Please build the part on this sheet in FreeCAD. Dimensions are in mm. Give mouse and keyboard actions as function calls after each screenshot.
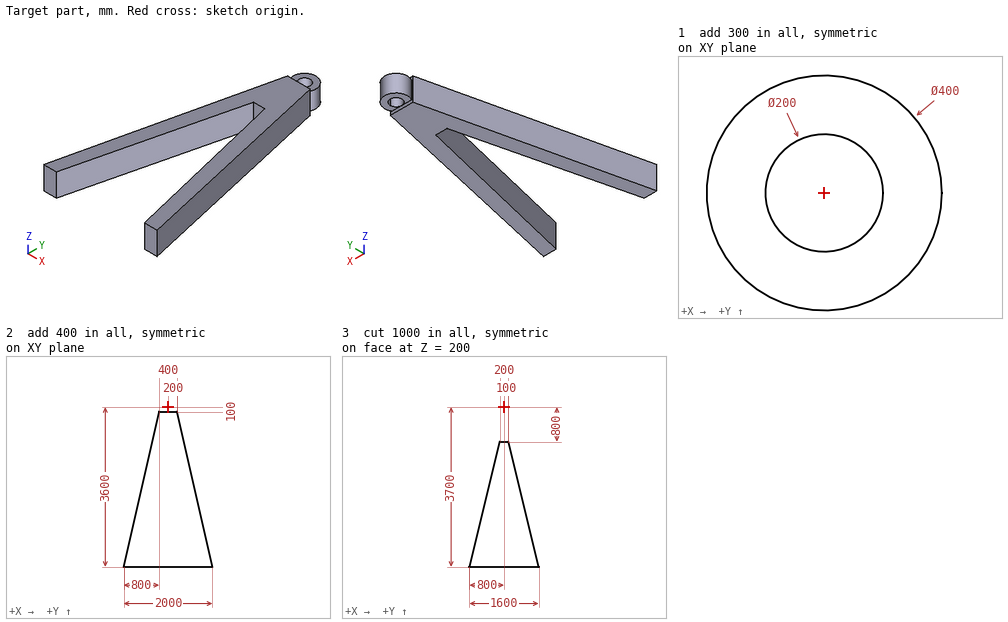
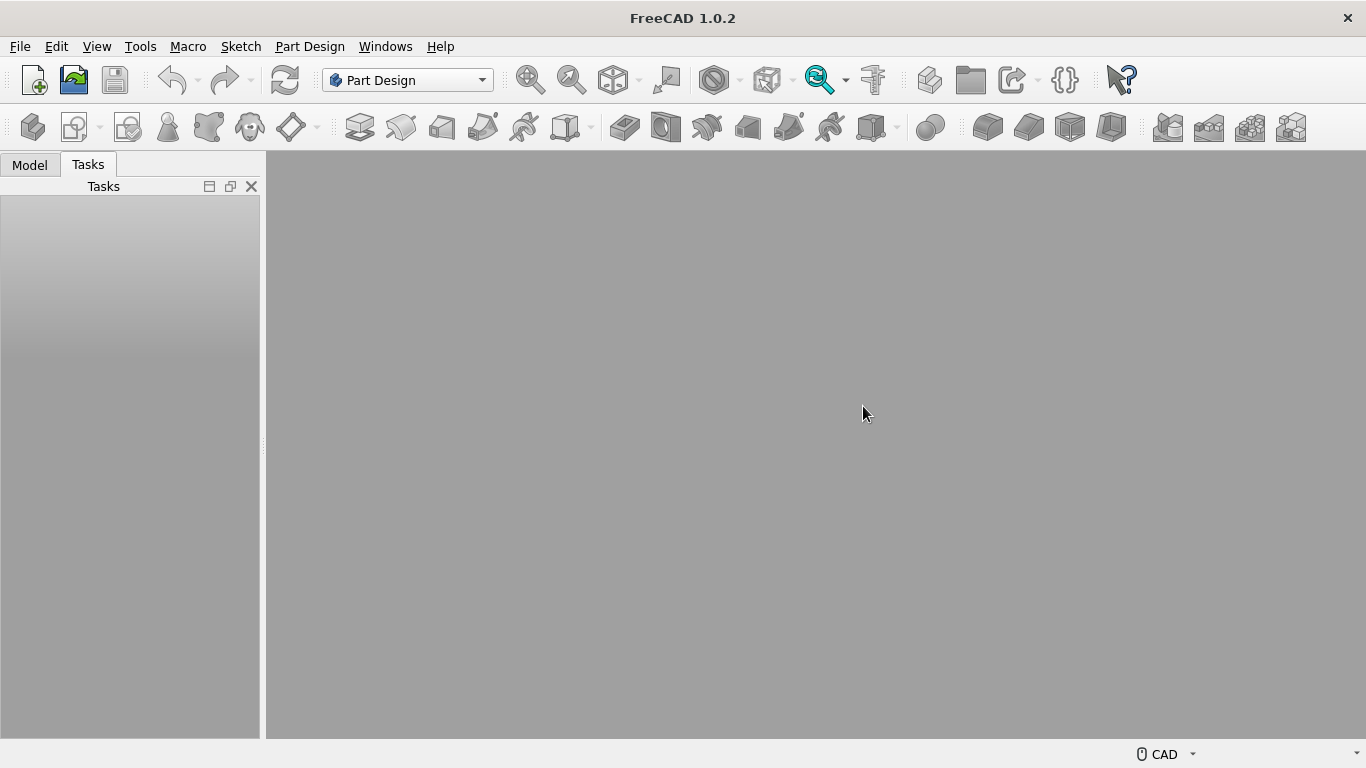
click(33, 80)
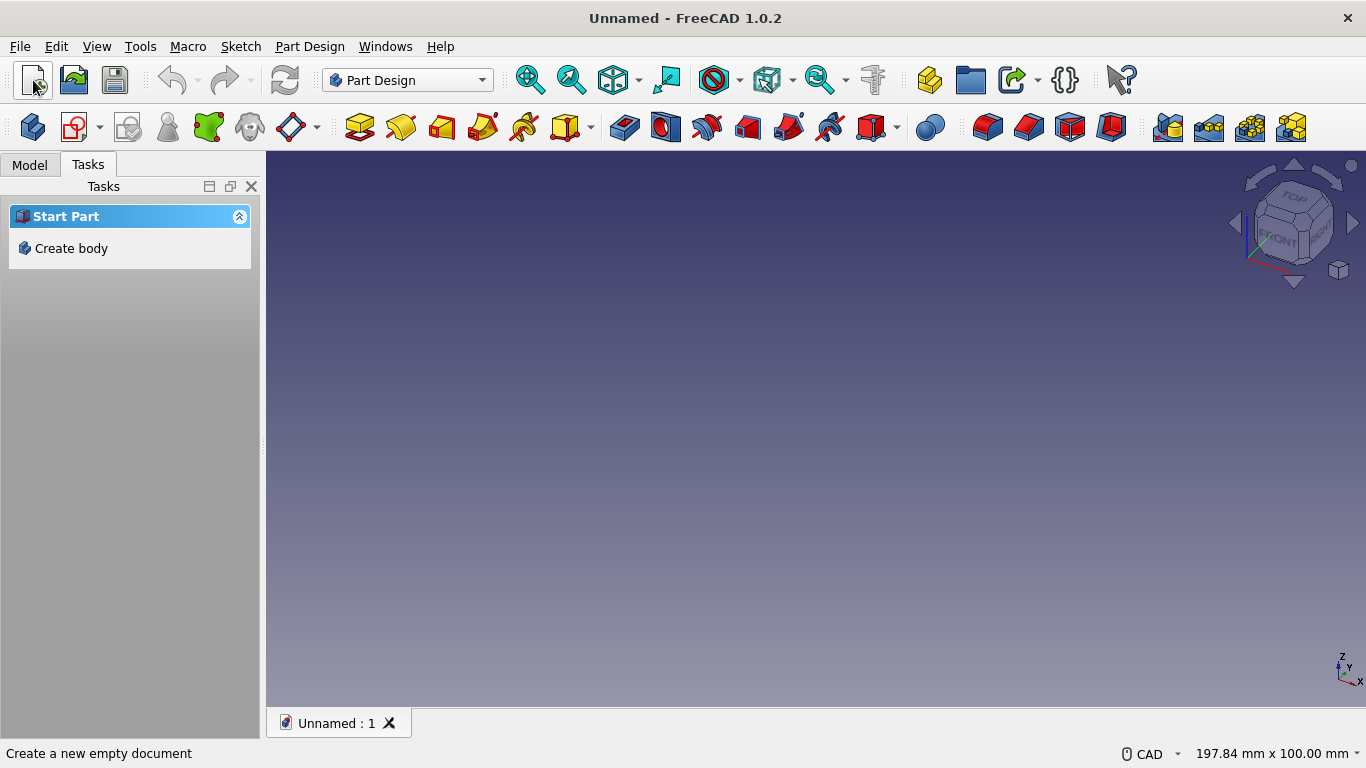
click(74, 128)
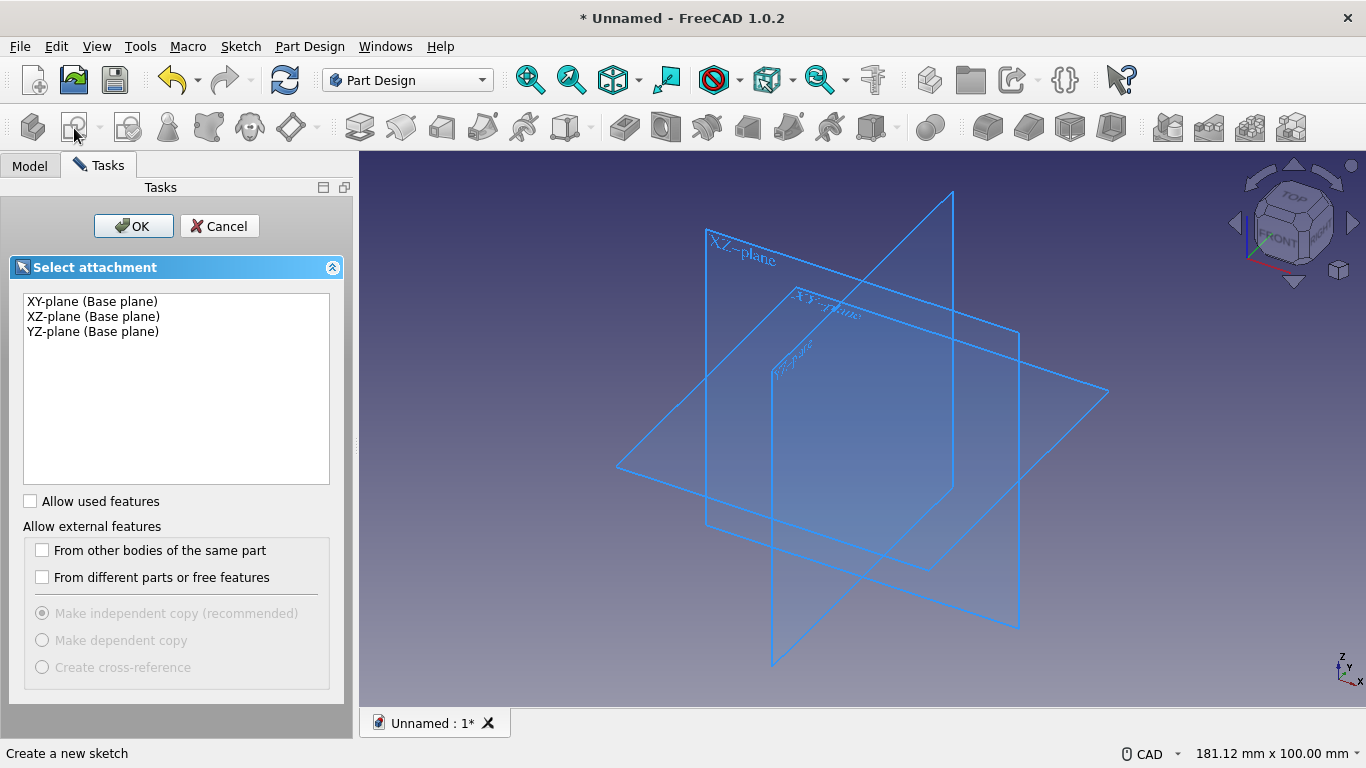
click(84, 302)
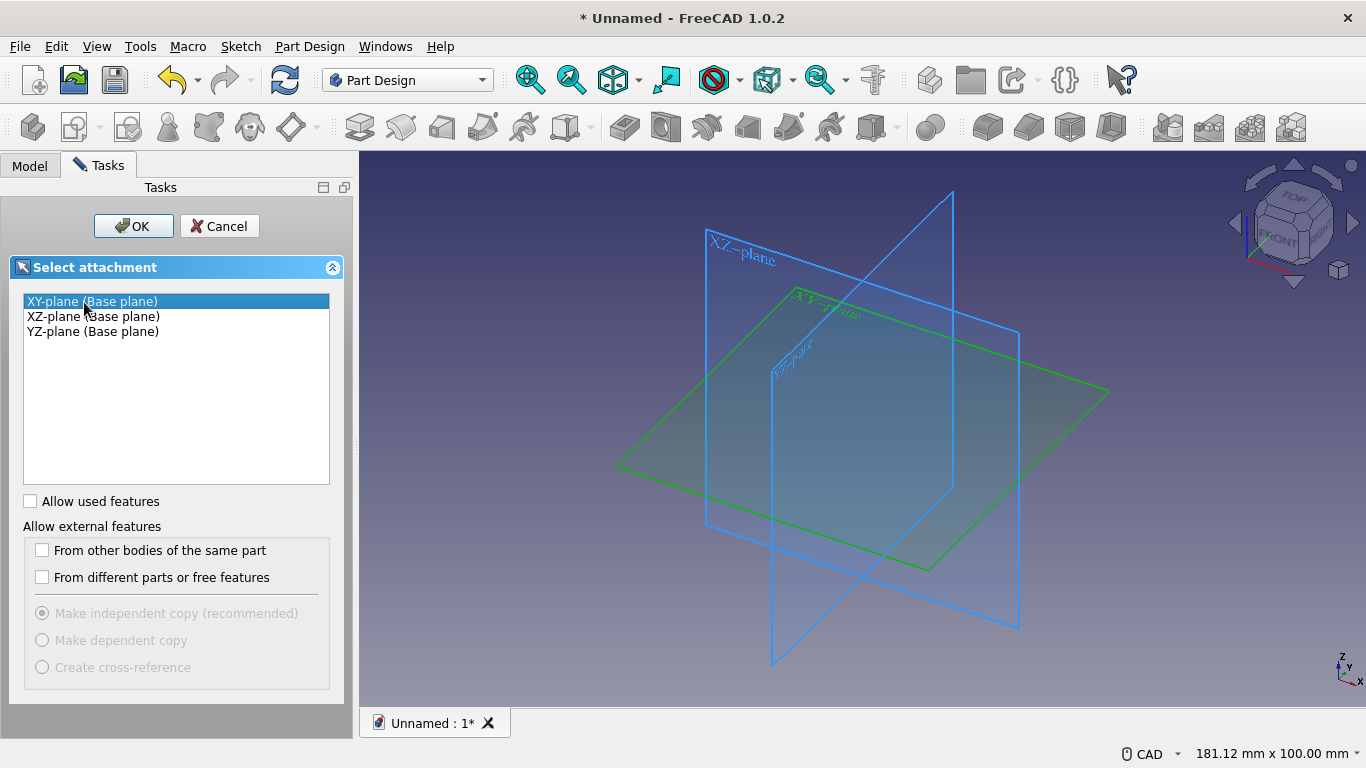
click(134, 226)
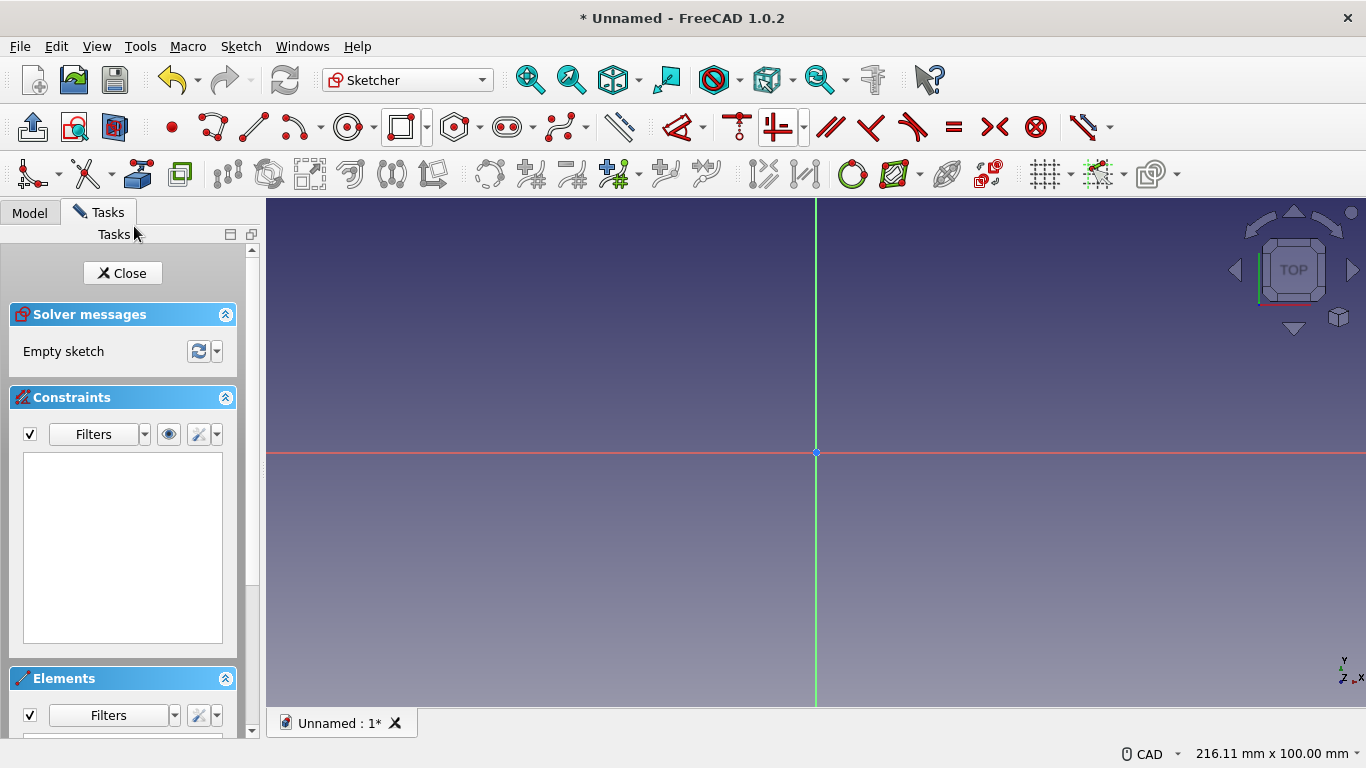
scroll(734, 452, down, 9)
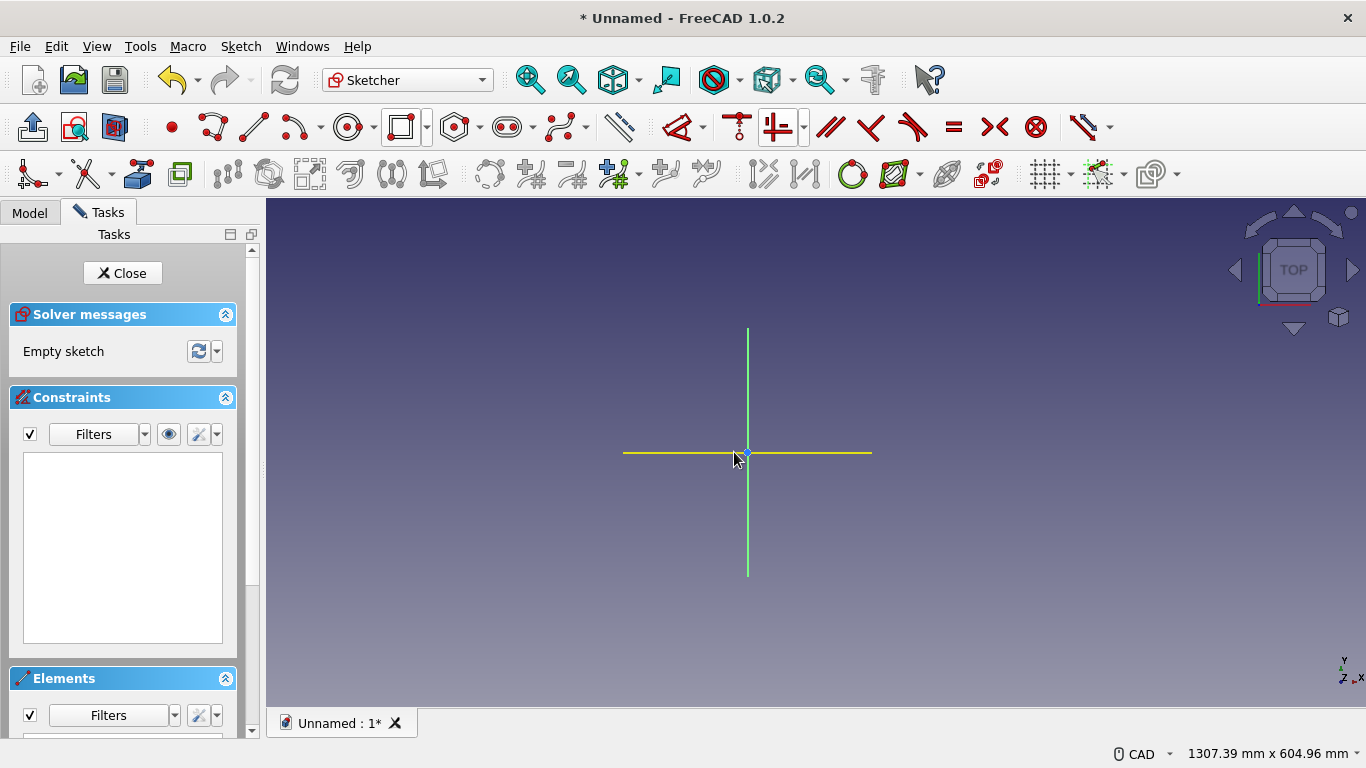
click(348, 128)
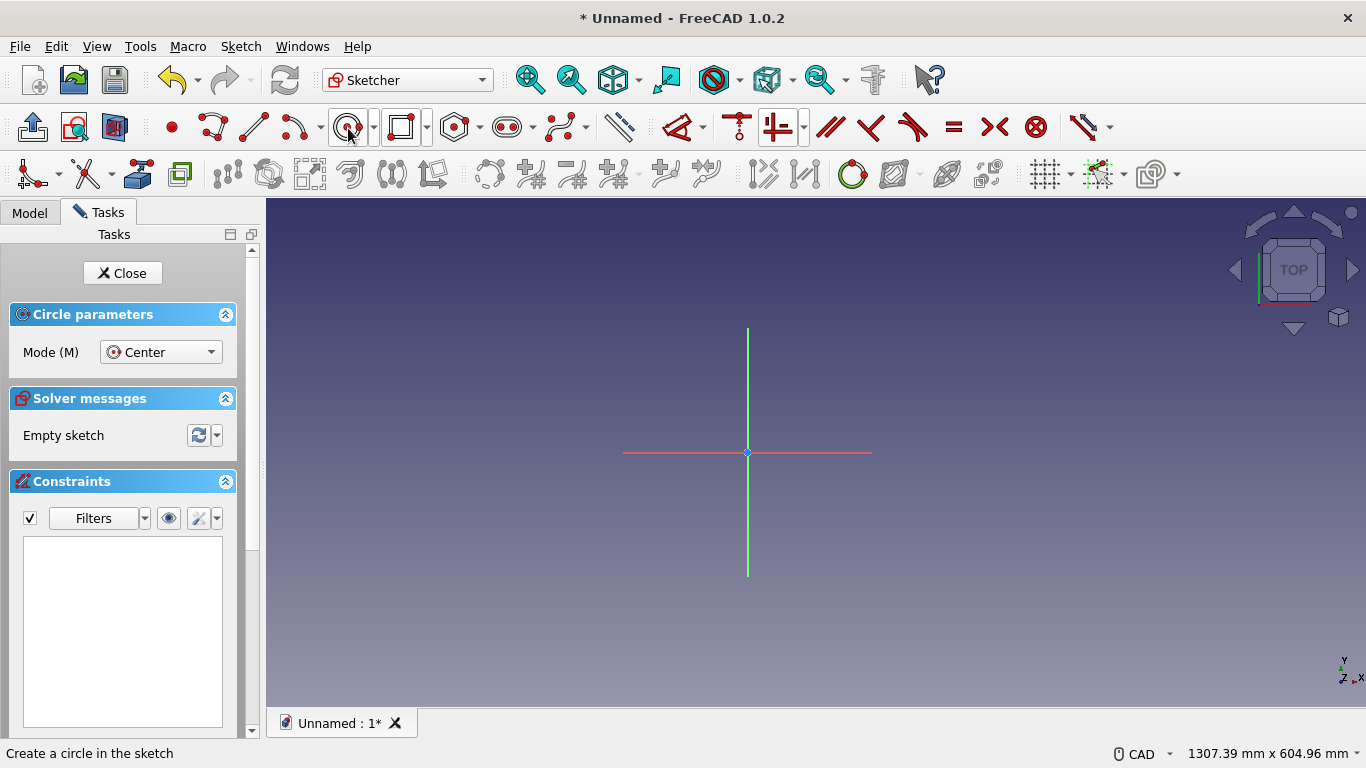
click(748, 452)
move(867, 334)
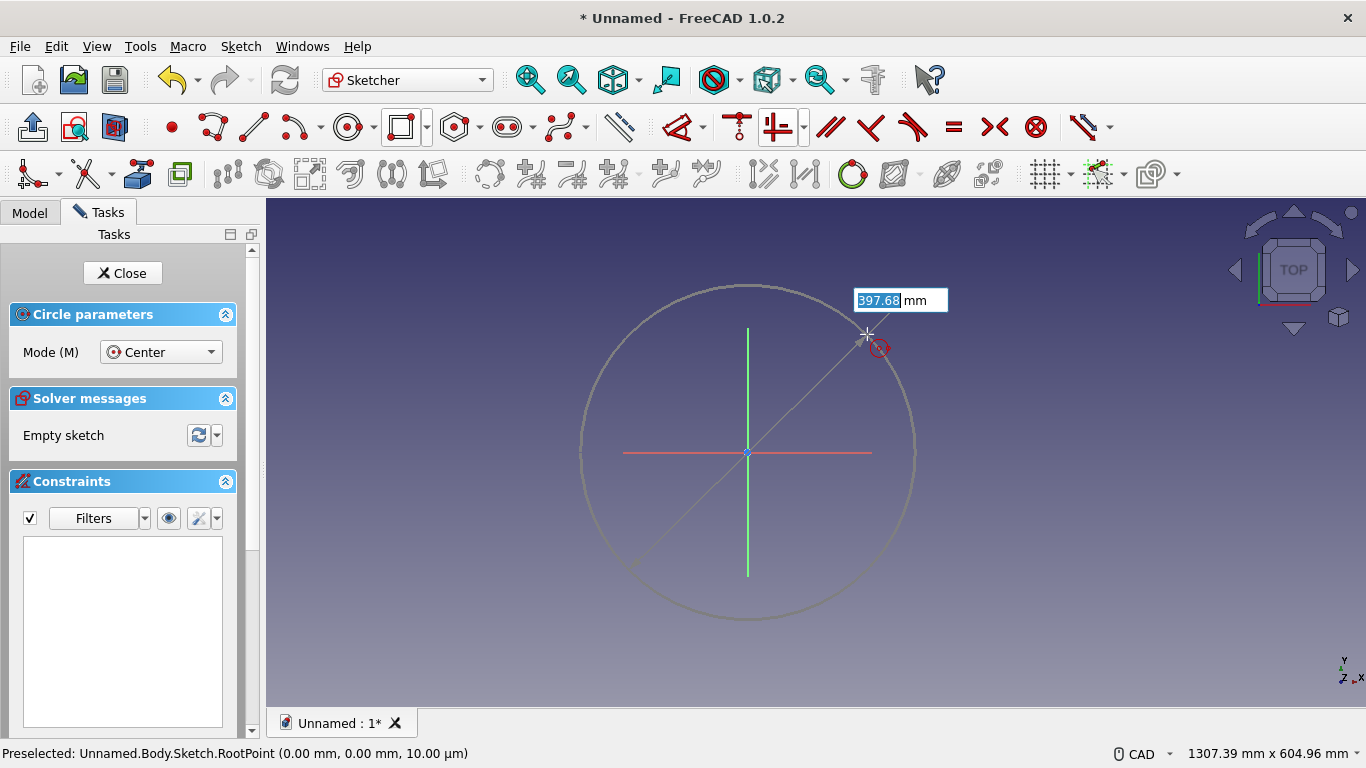
text(400)
key(Return)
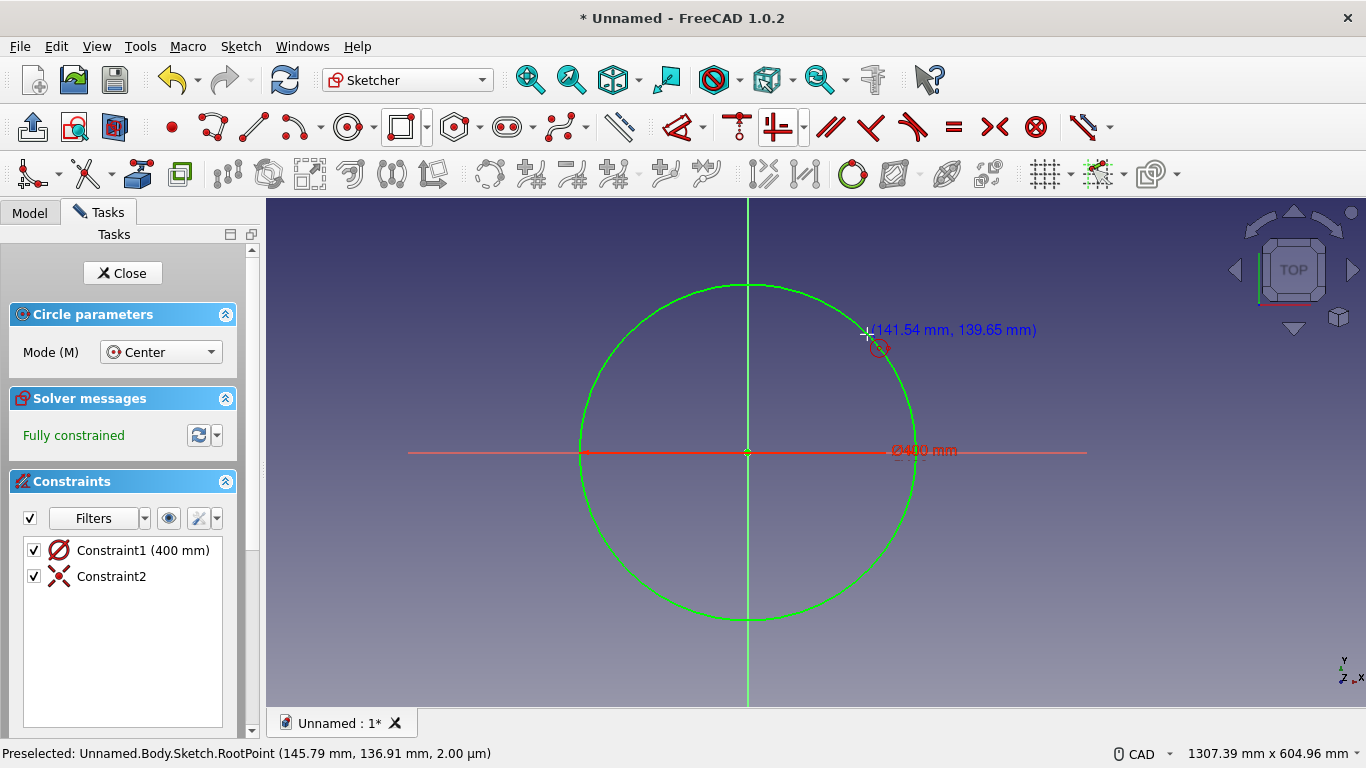
click(748, 452)
move(807, 393)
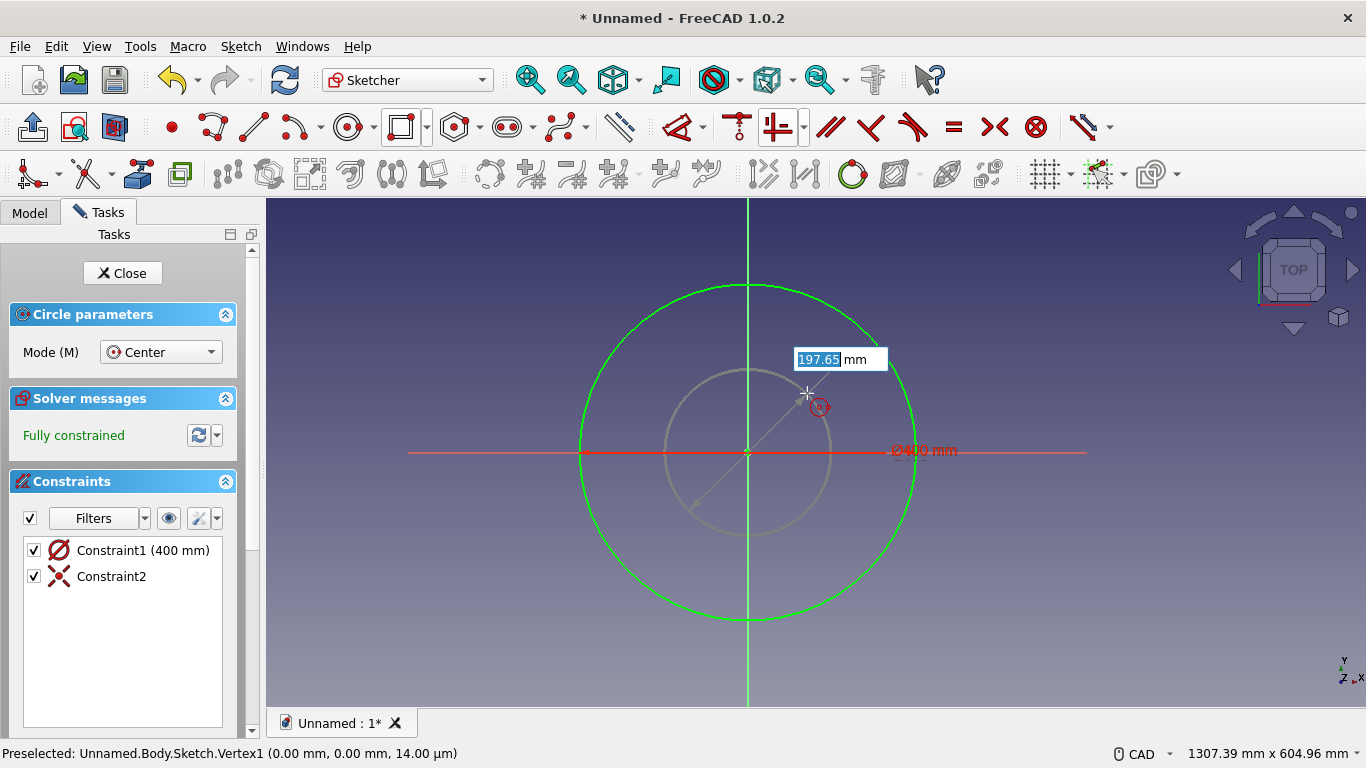
text(200)
key(Return)
key(Escape)